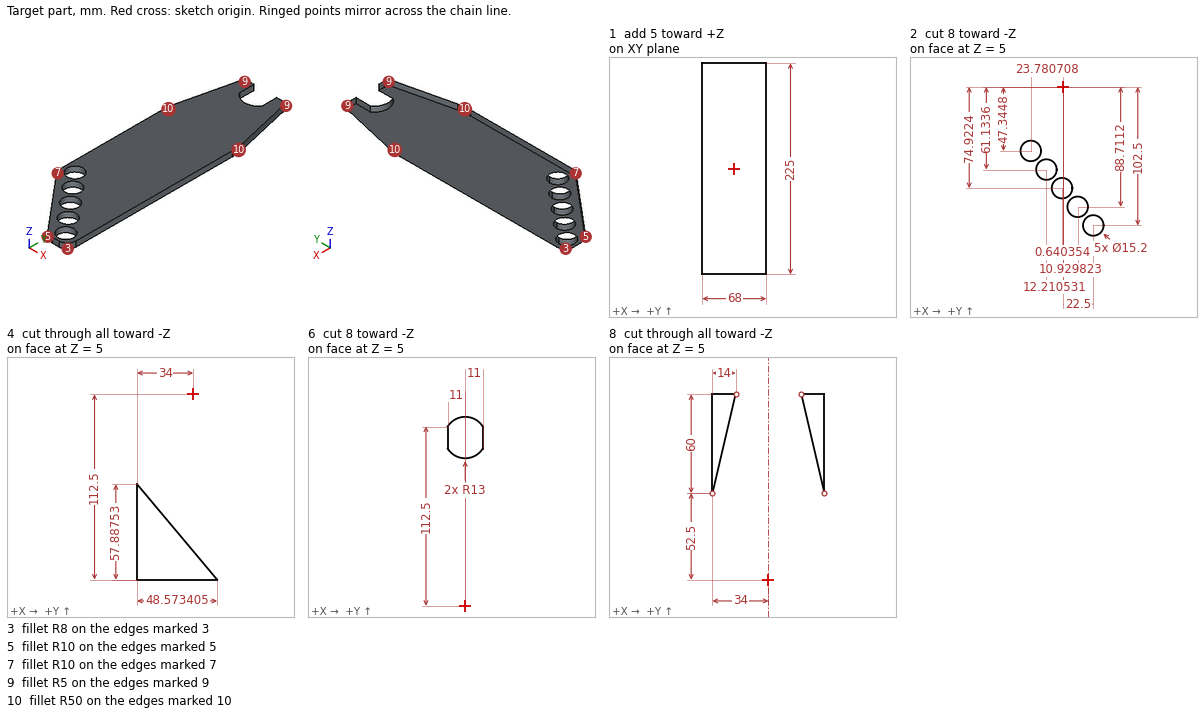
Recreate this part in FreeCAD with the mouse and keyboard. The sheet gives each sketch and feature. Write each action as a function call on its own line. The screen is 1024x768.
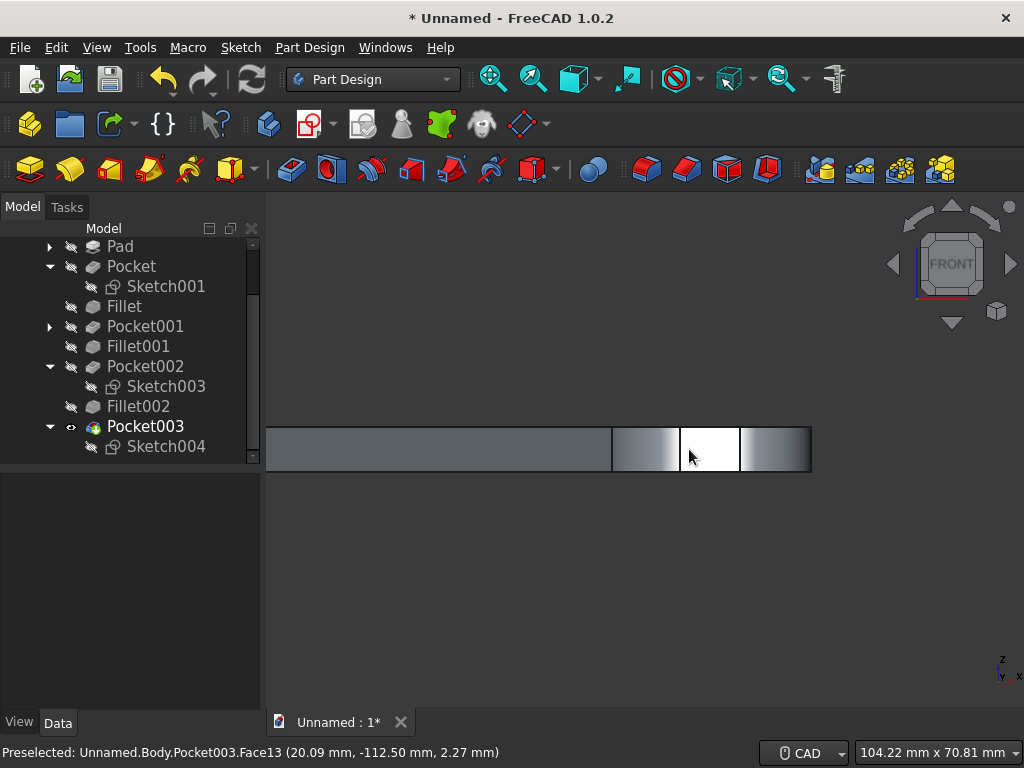
click(494, 80)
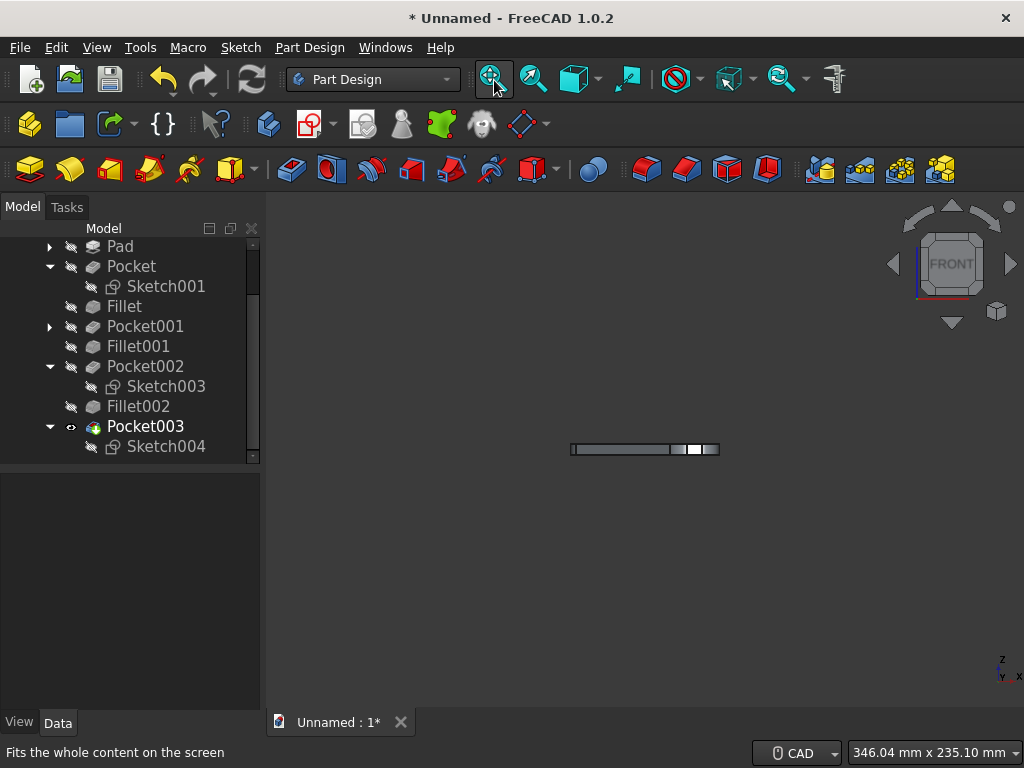
key(3)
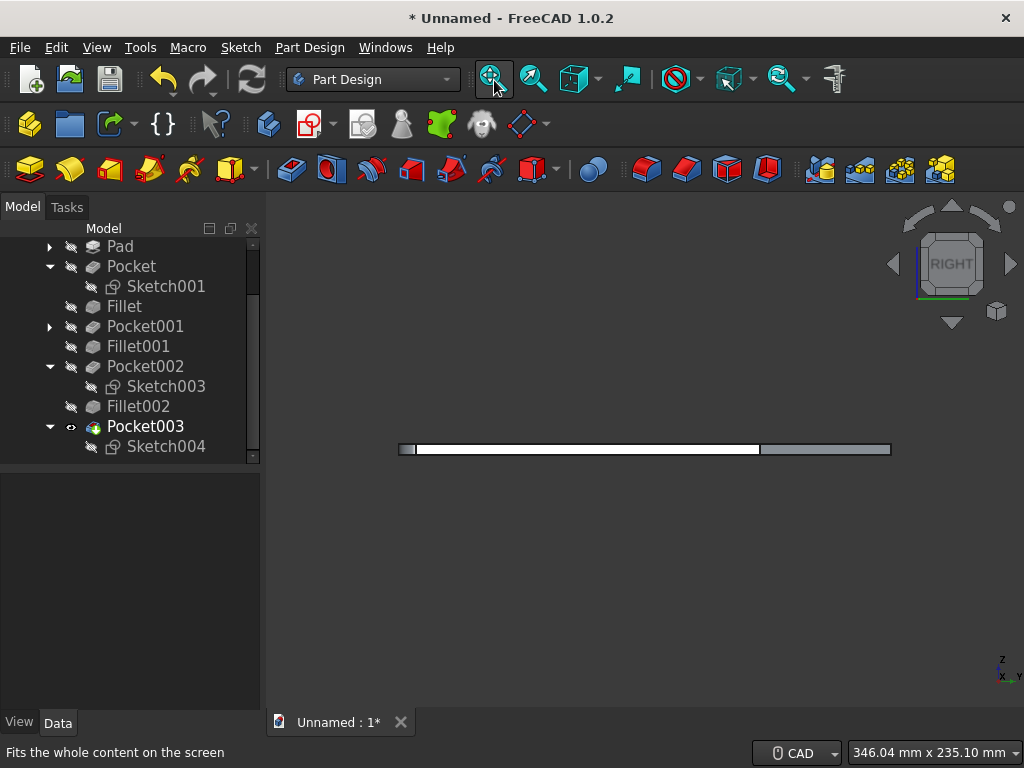
key(5)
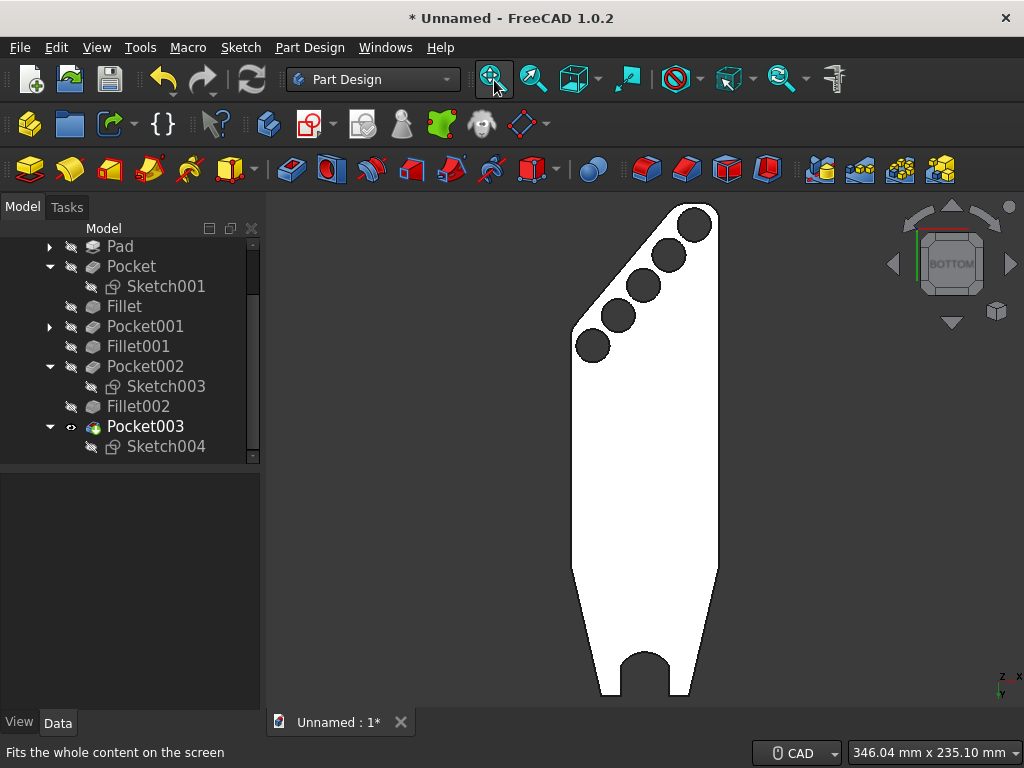
key(4)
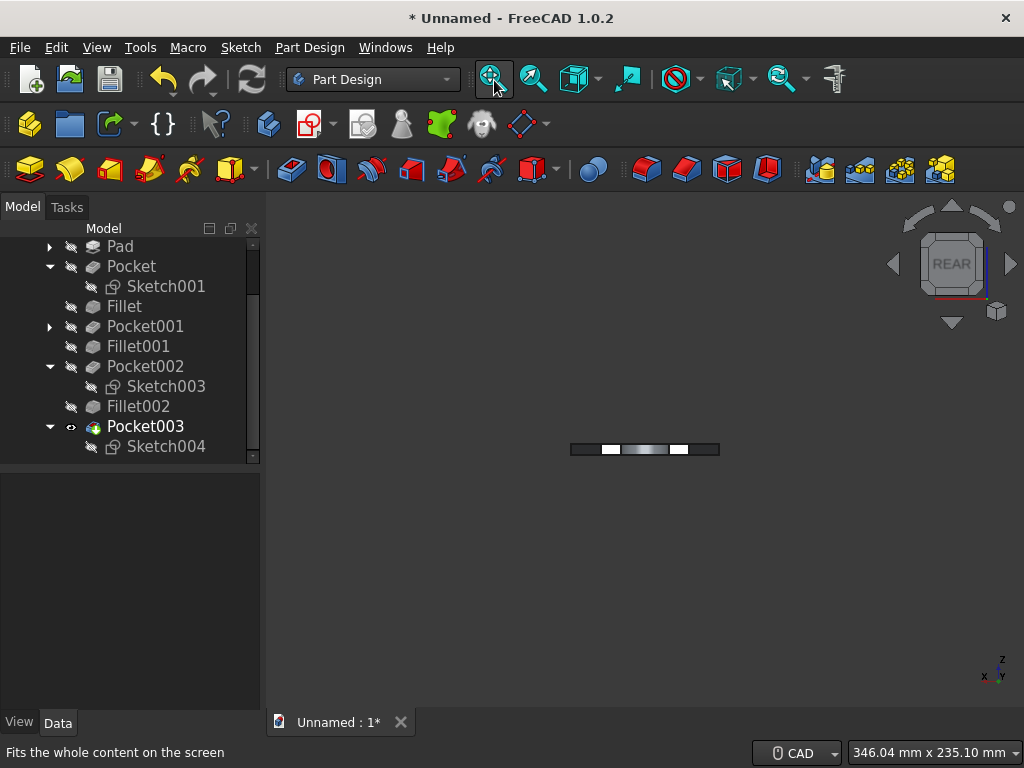
key(v)
key(f)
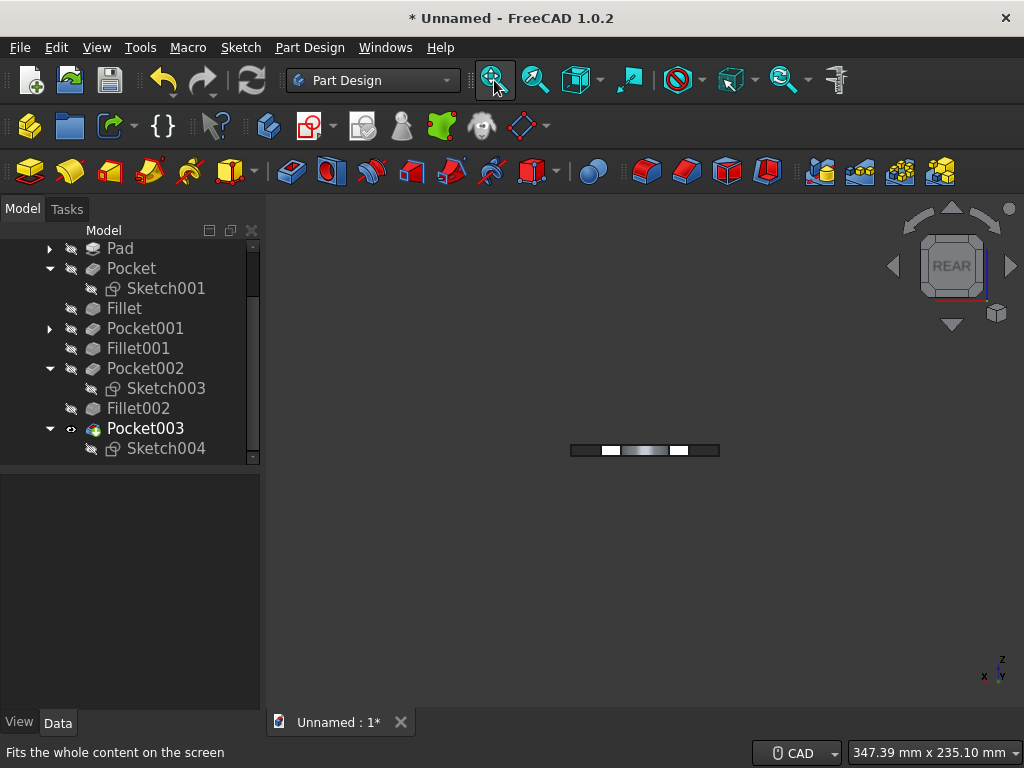
scroll(601, 450, up, 7)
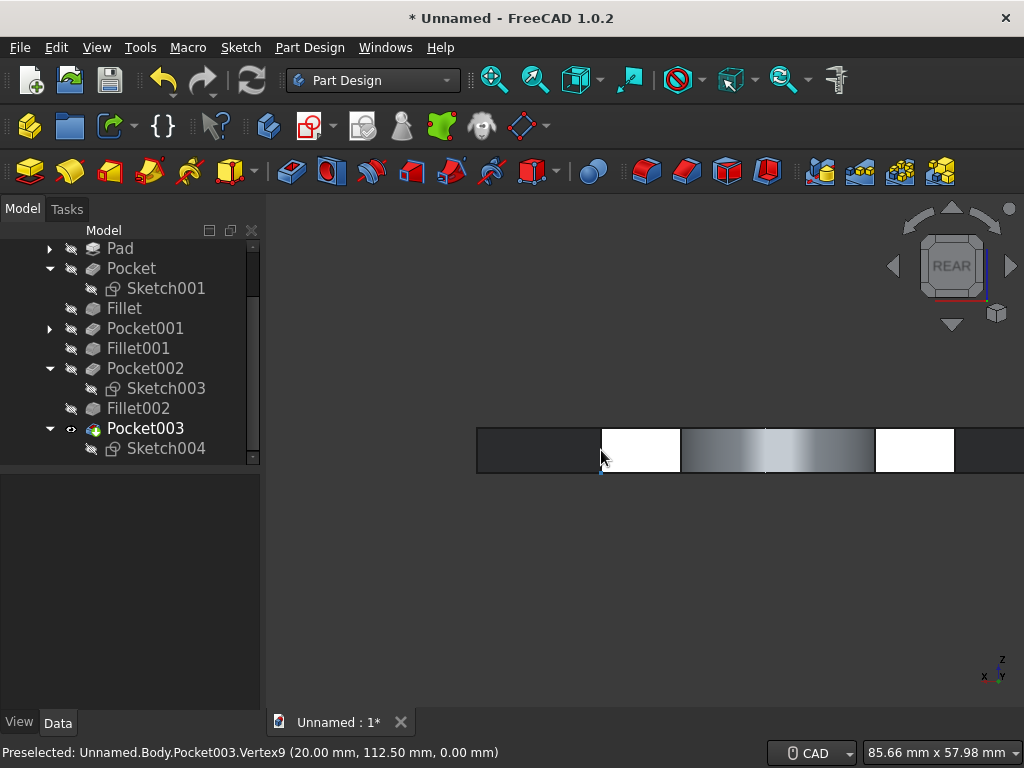
click(601, 450)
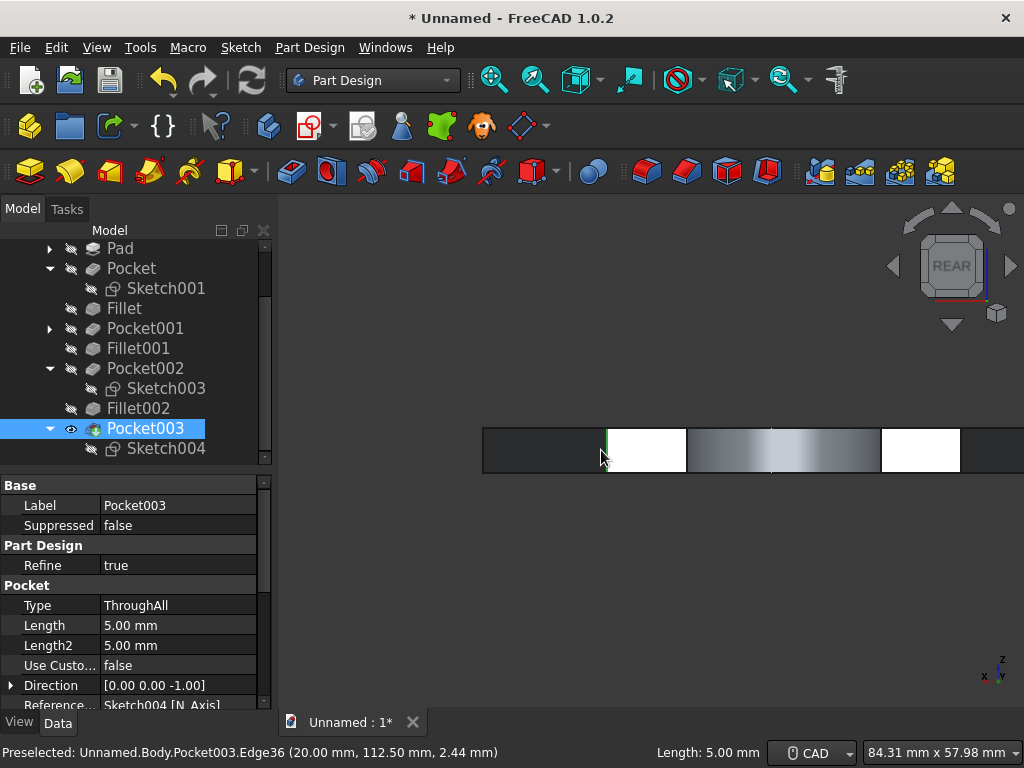
click(496, 80)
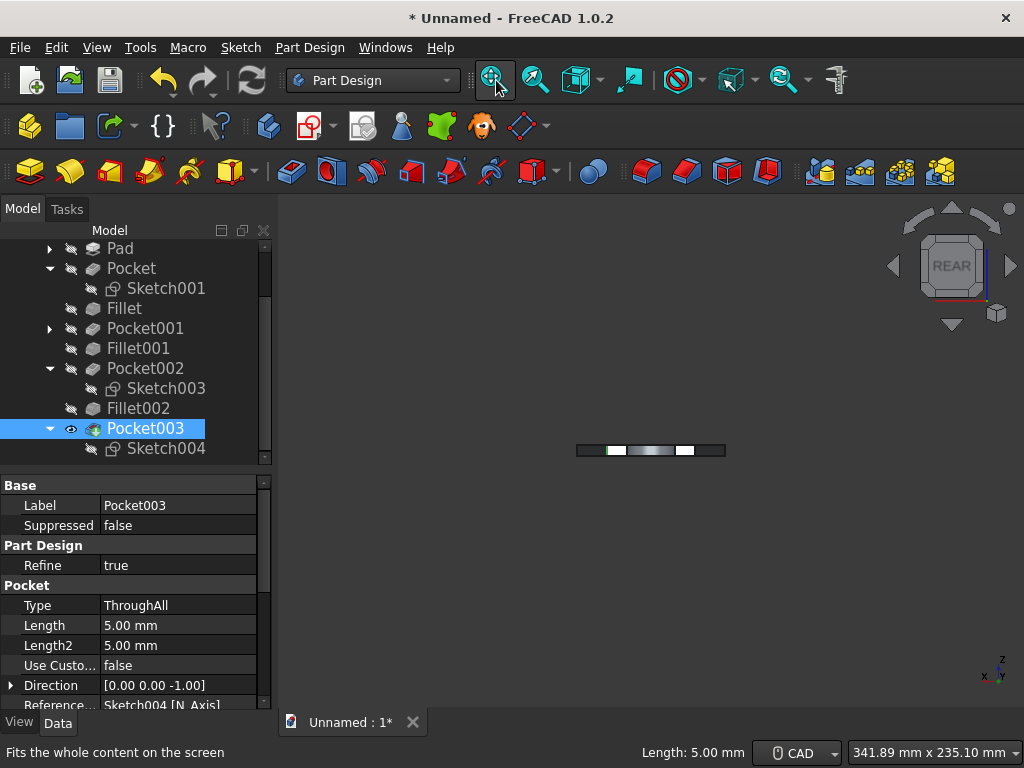
key(6)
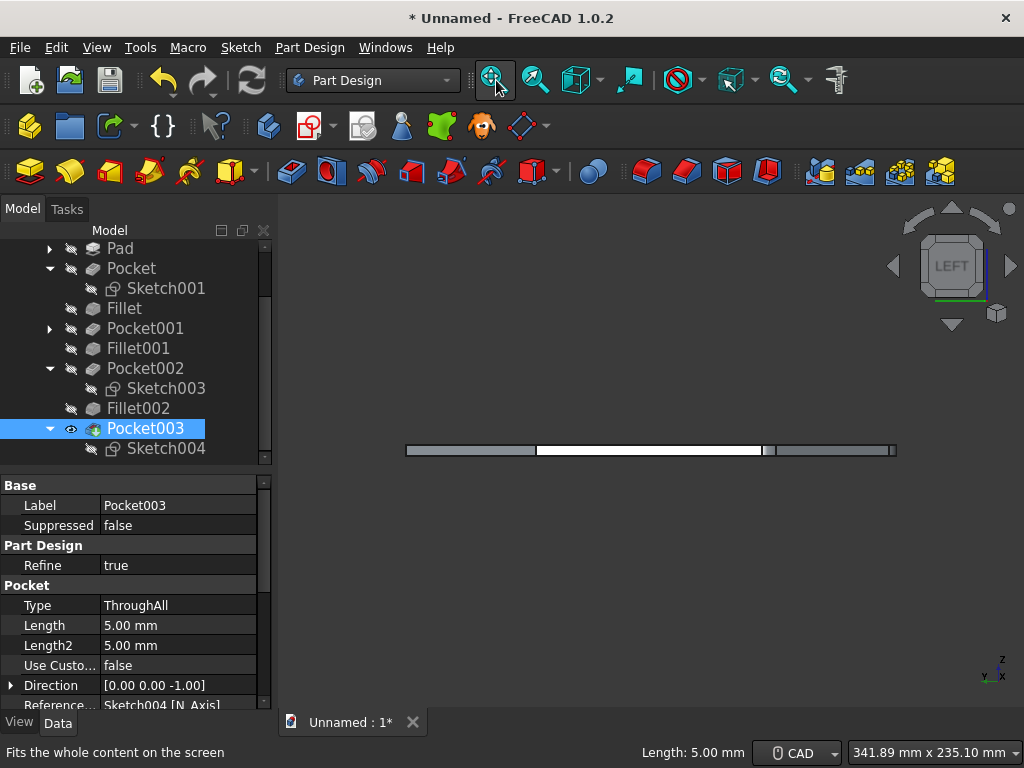
scroll(406, 449, up, 7)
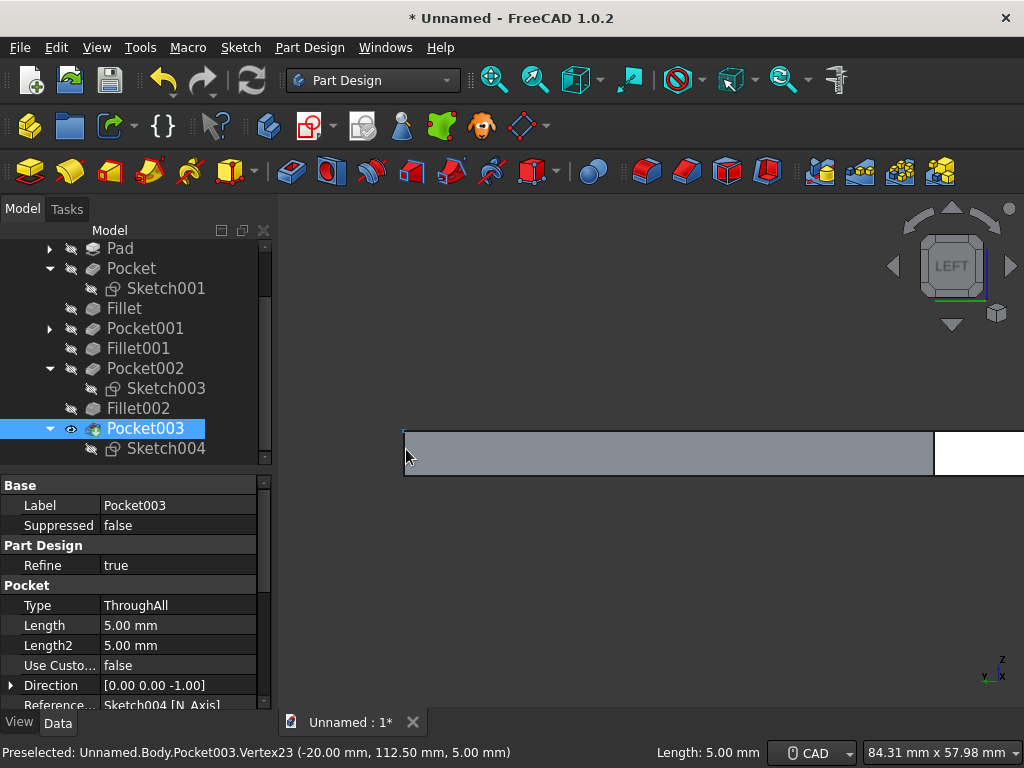
click(496, 80)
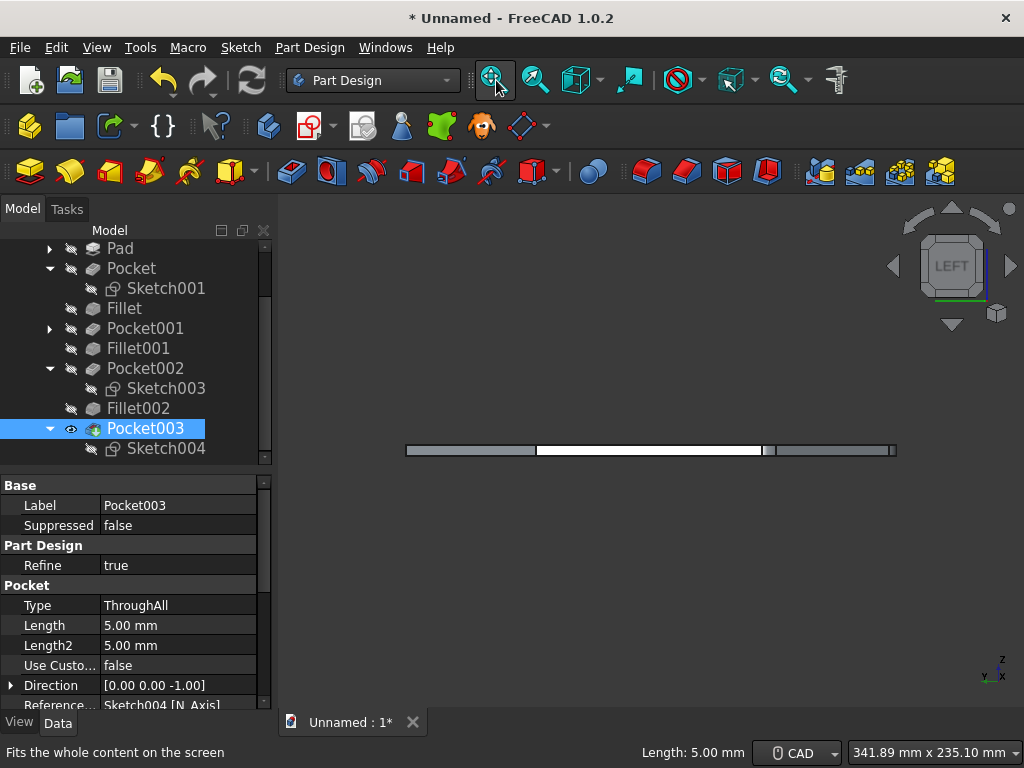
key(v)
key(3)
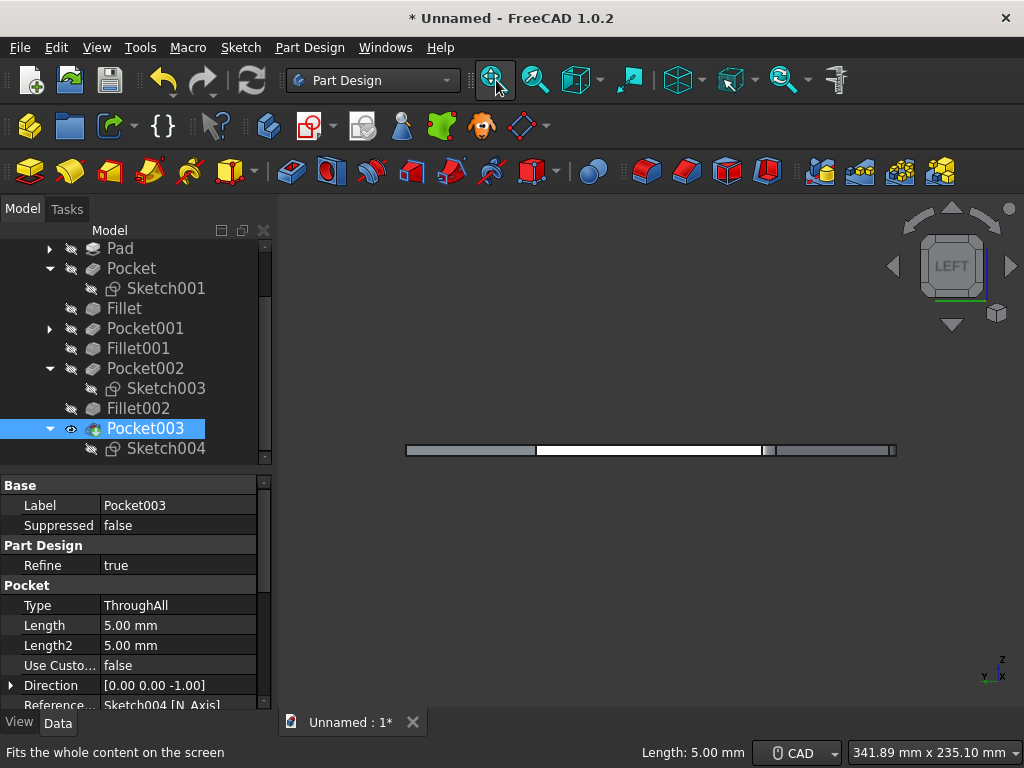
key(0)